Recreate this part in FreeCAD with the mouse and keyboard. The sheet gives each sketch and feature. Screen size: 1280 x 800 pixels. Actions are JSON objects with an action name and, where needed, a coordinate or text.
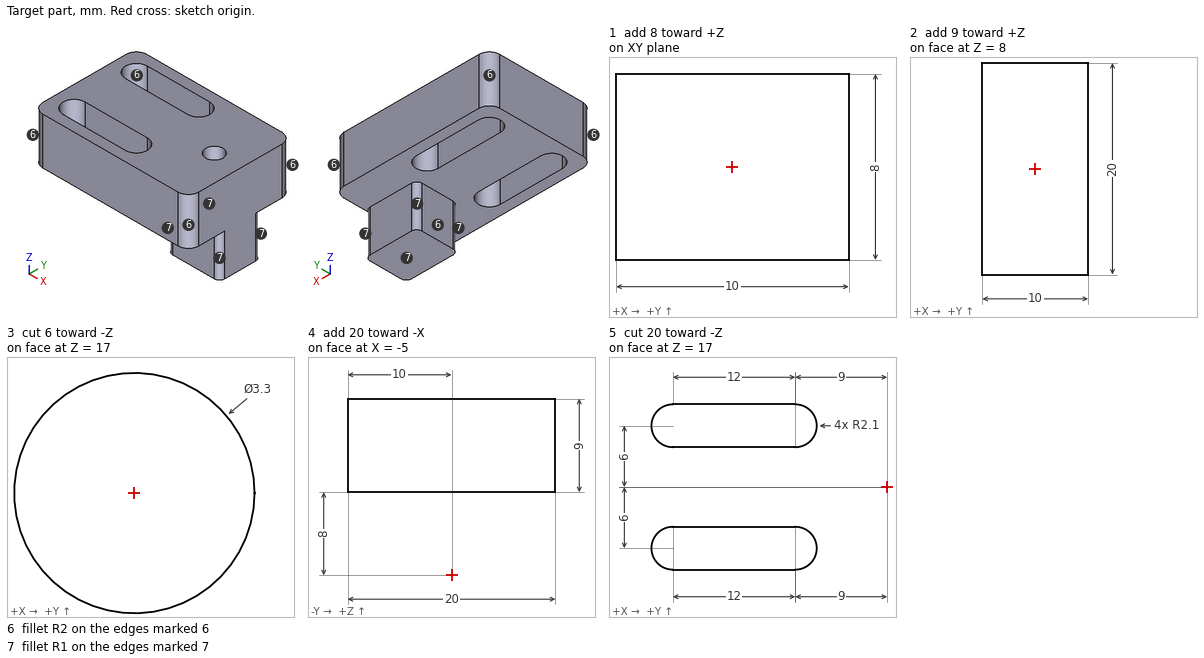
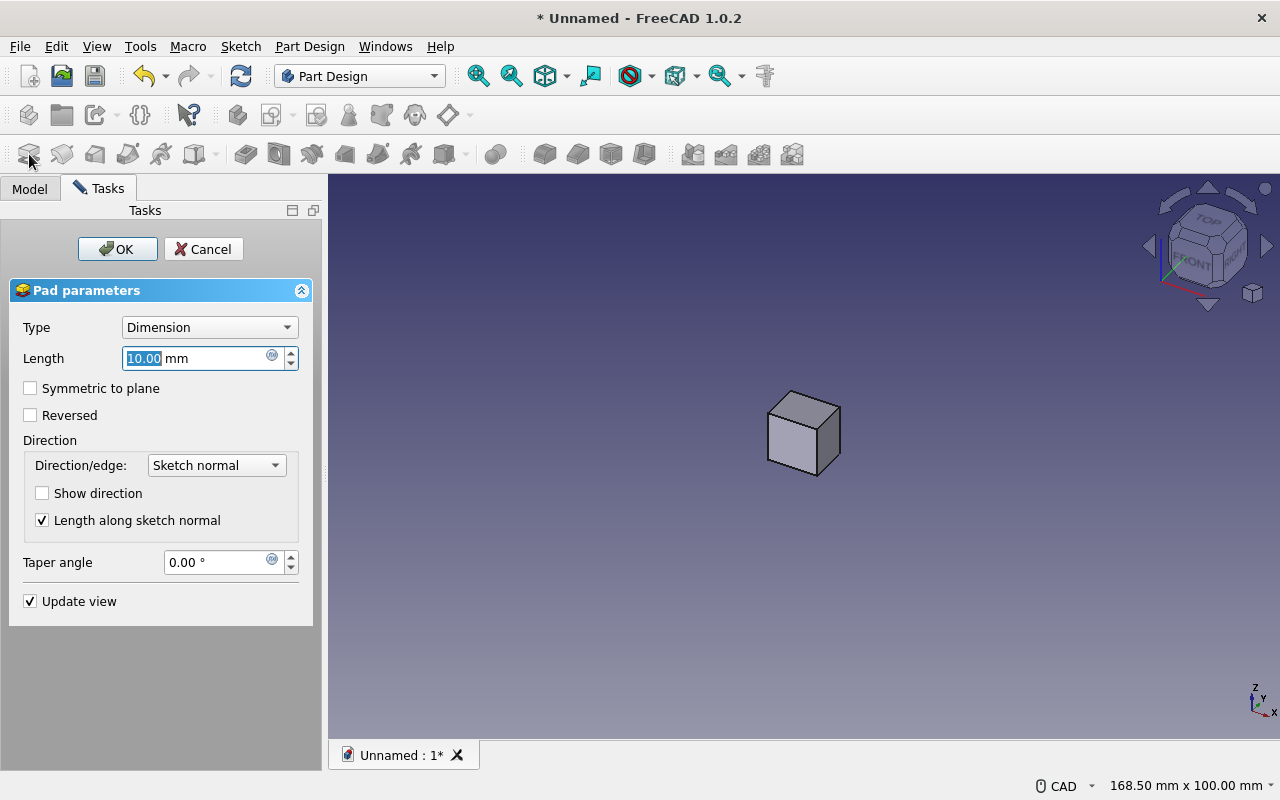
{"action": "type", "text": "8"}
{"action": "key", "text": "Tab"}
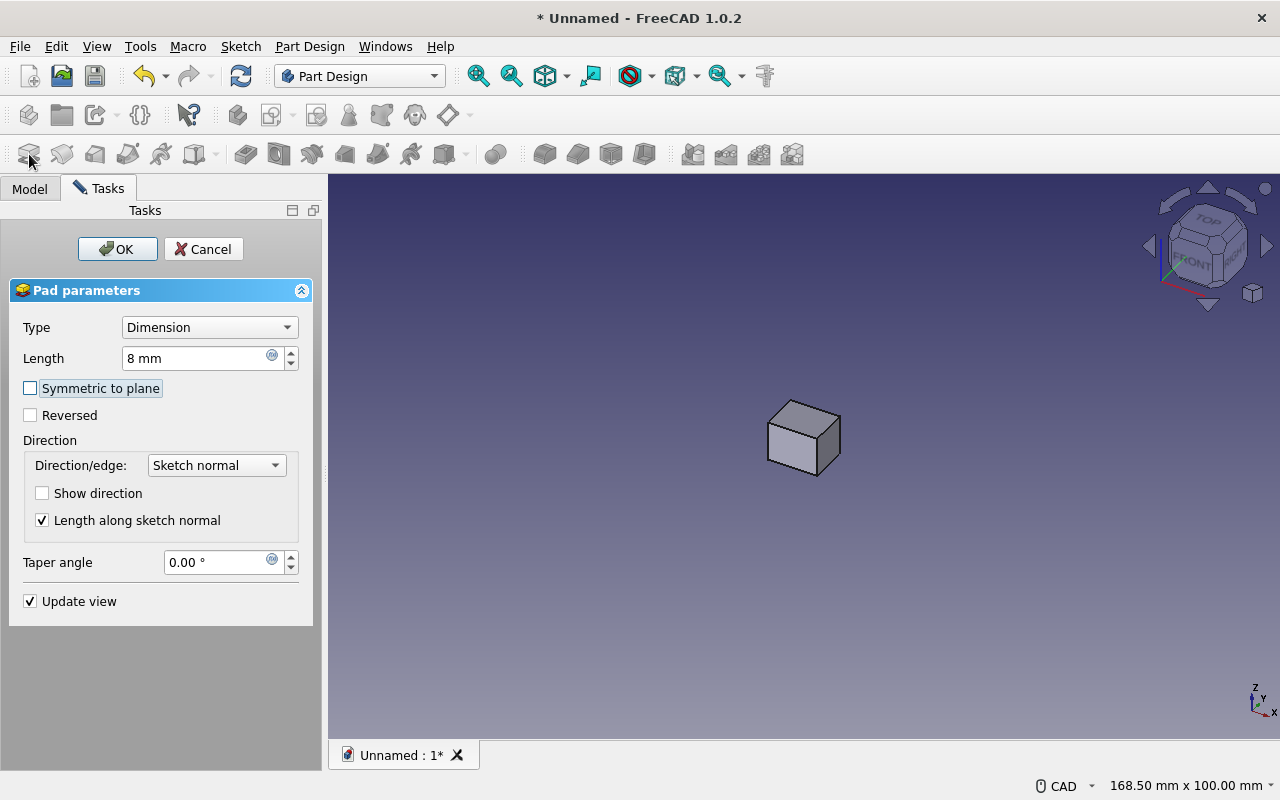
{"action": "left_click", "coordinate": [118, 249]}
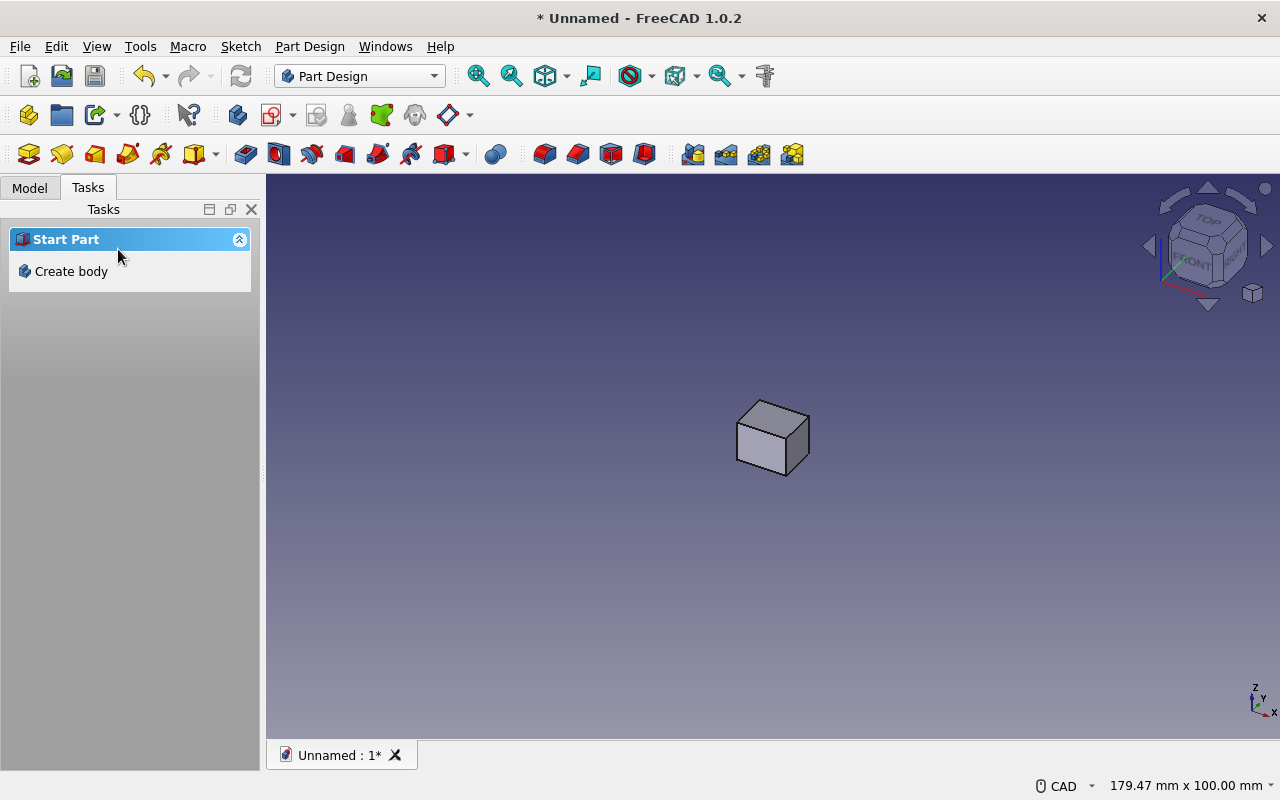
{"action": "left_click", "coordinate": [479, 76]}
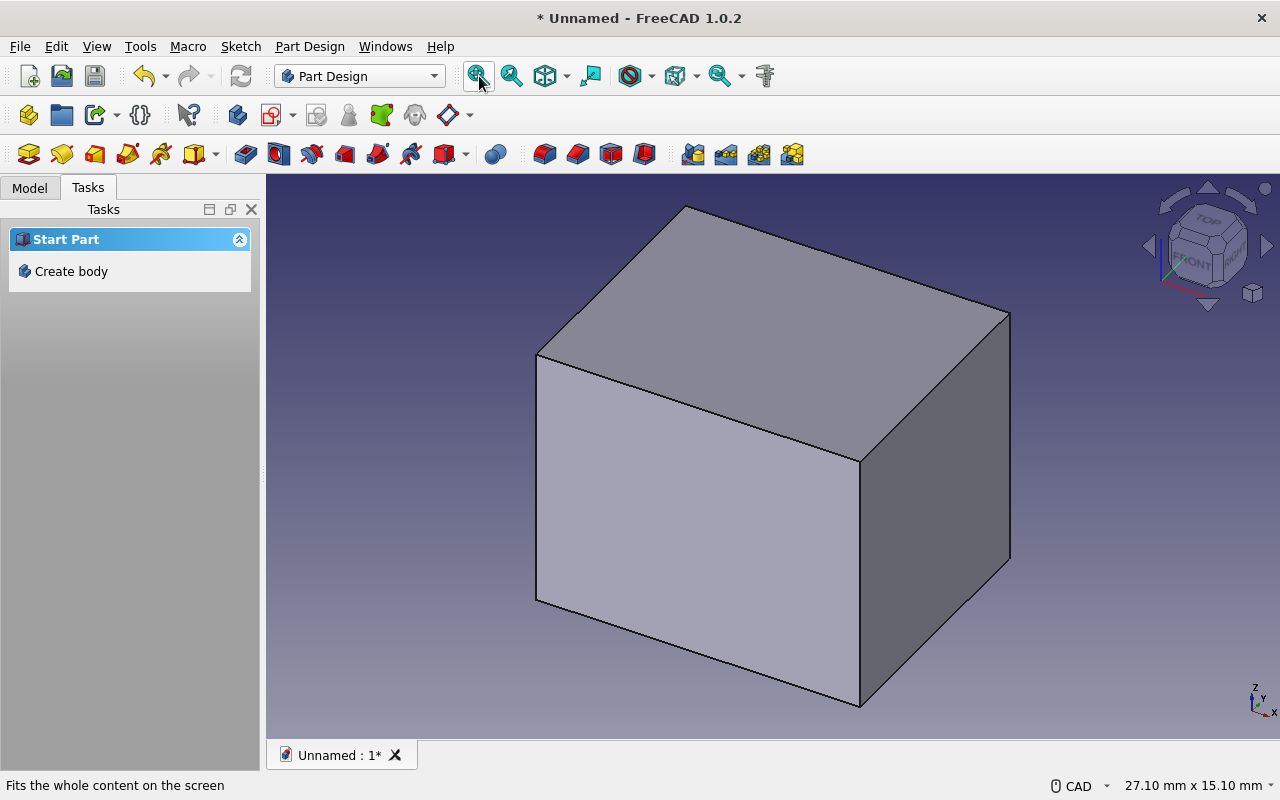
{"action": "left_click", "coordinate": [773, 333]}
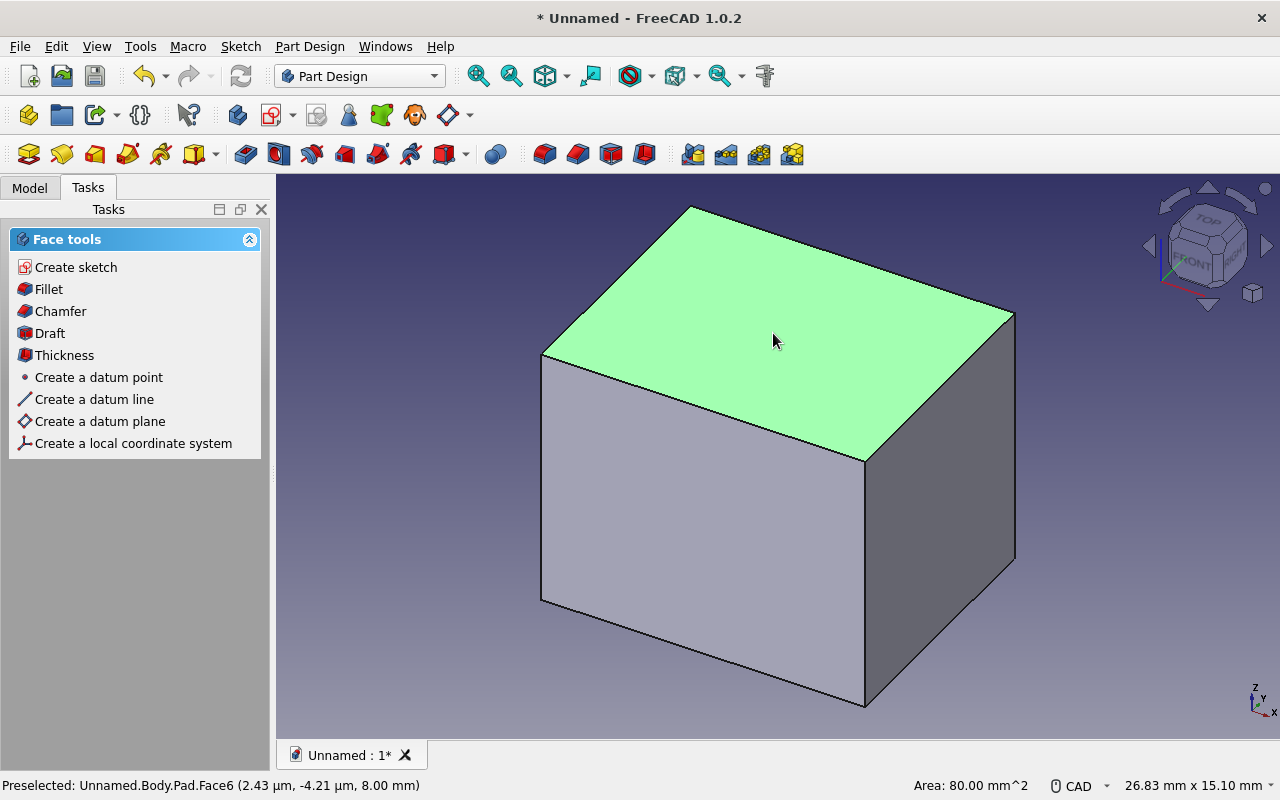
{"action": "left_click", "coordinate": [270, 116]}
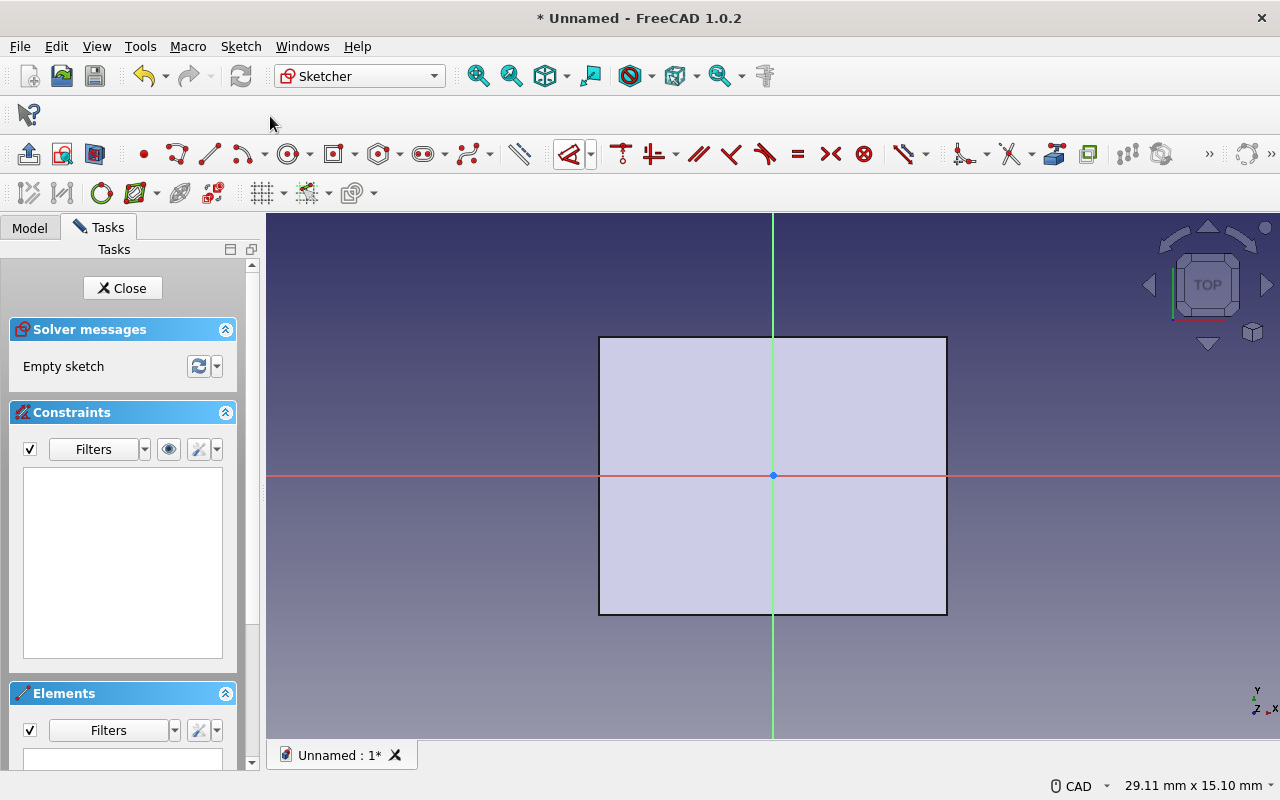
{"action": "scroll", "coordinate": [649, 476], "scroll_direction": "down", "scroll_amount": 4}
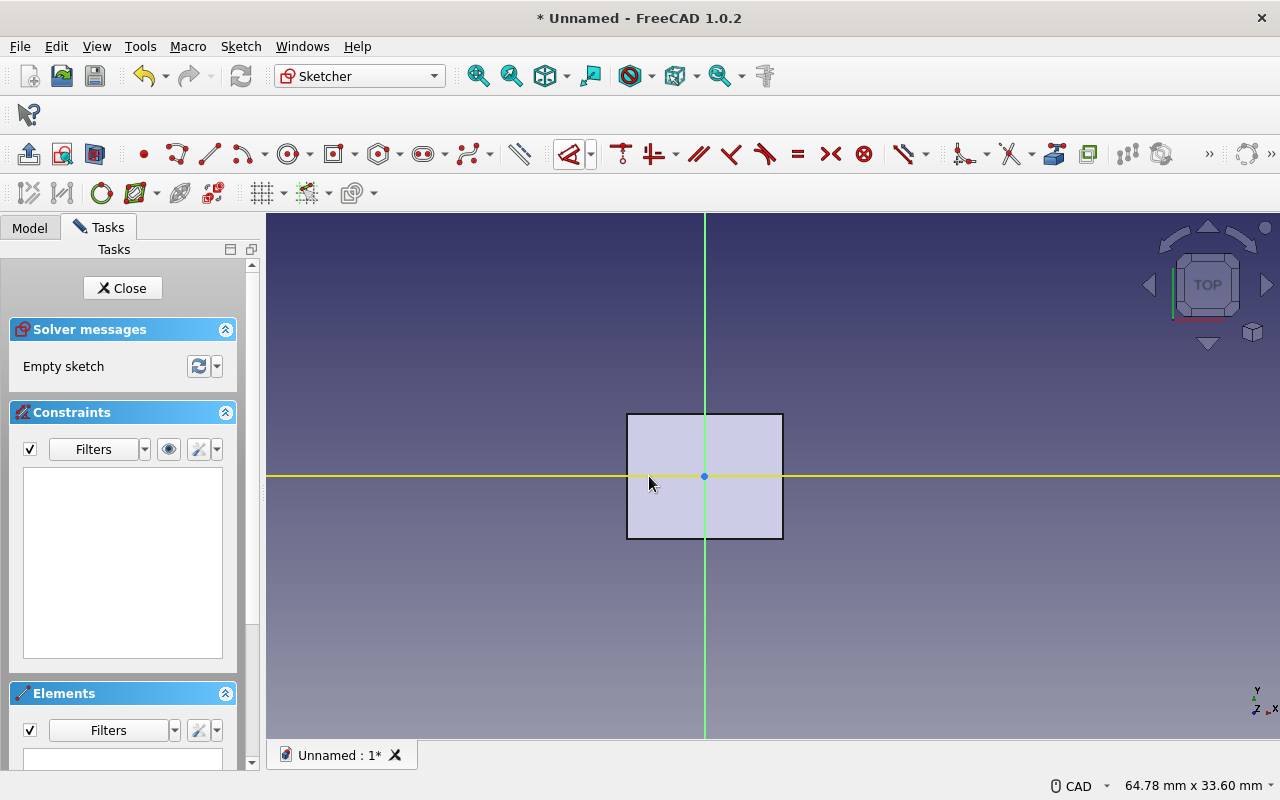
{"action": "left_click", "coordinate": [332, 154]}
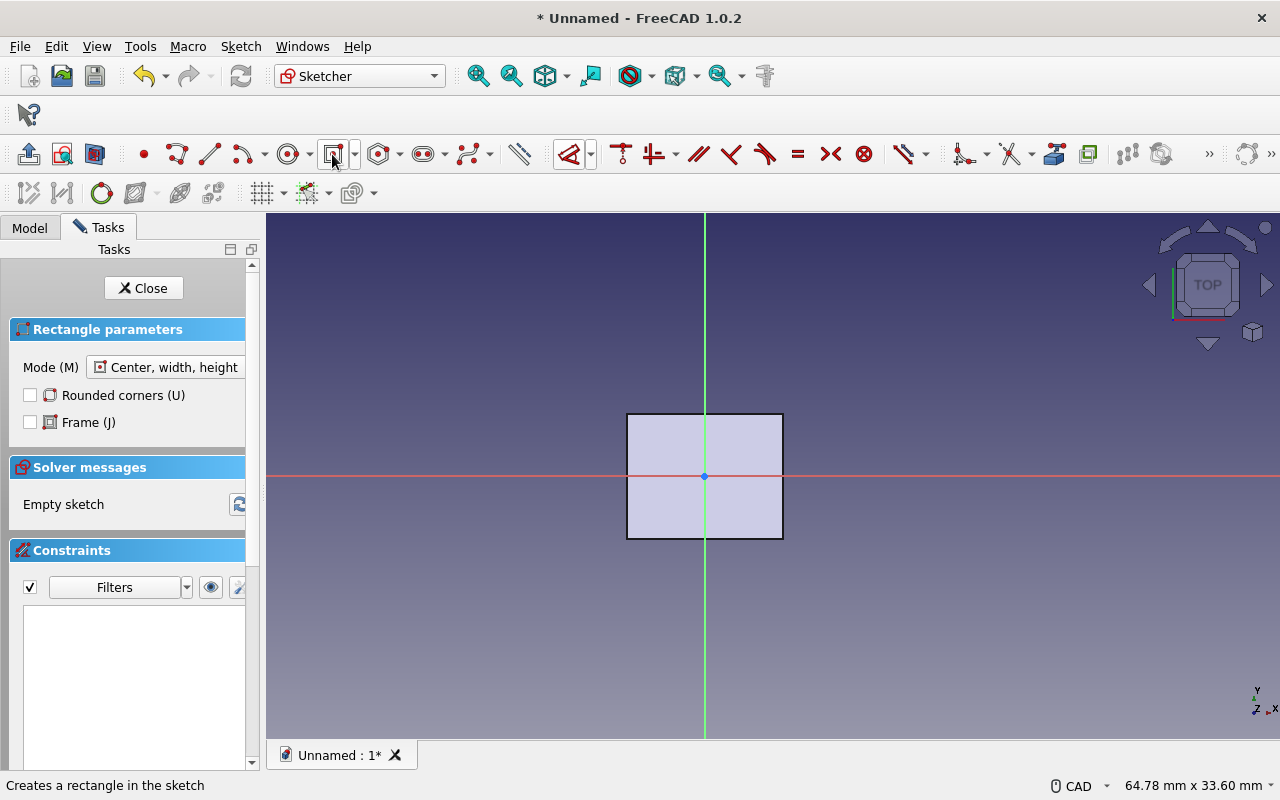
{"action": "left_click", "coordinate": [705, 476]}
{"action": "mouse_move", "coordinate": [783, 320]}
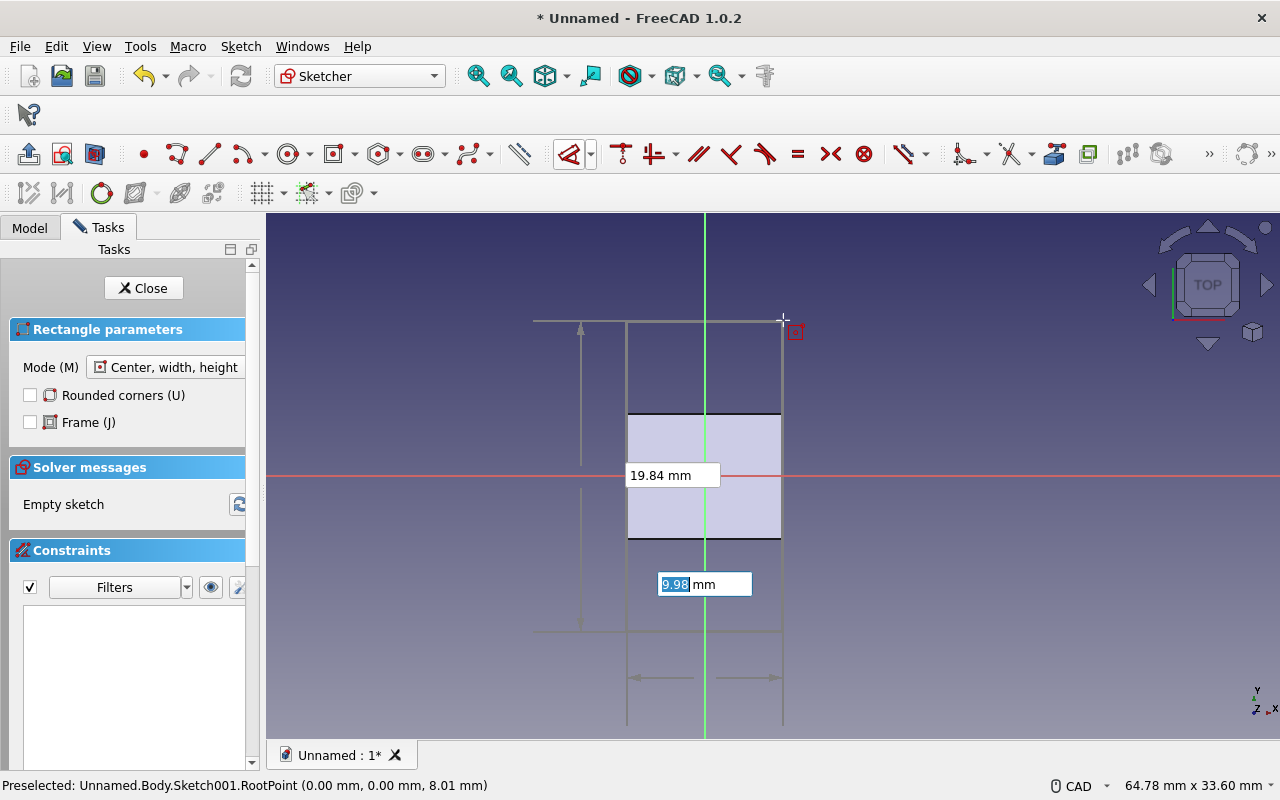
{"action": "type", "text": "10"}
{"action": "key", "text": "Tab"}
{"action": "type", "text": "20"}
{"action": "key", "text": "Return"}
{"action": "key", "text": "Escape"}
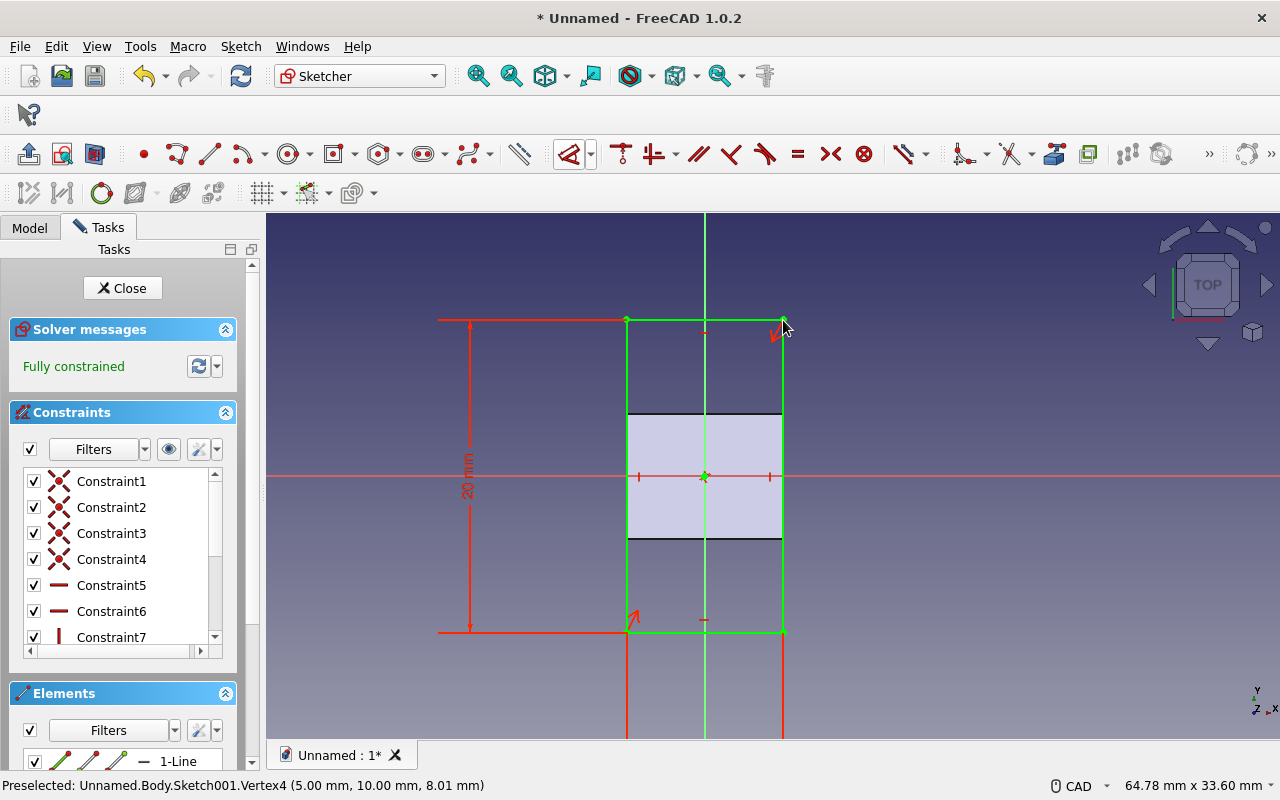
{"action": "left_click", "coordinate": [123, 288]}